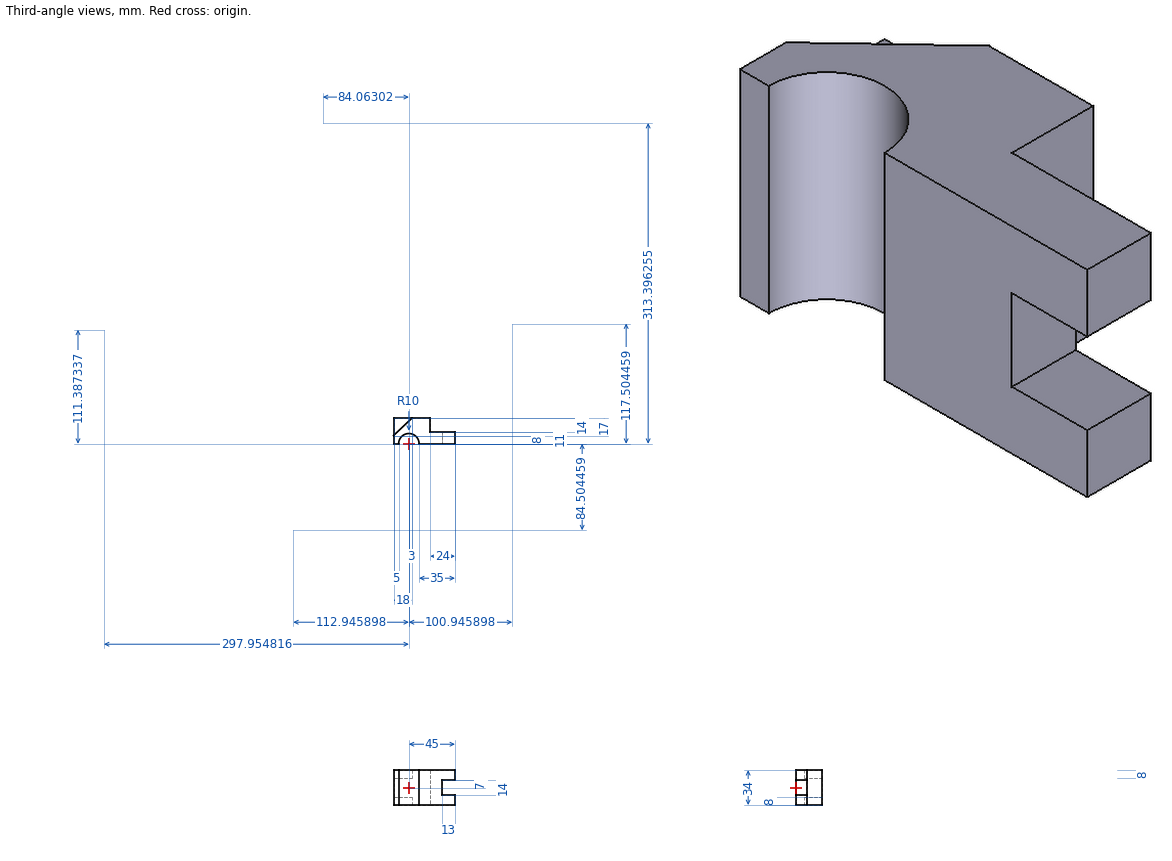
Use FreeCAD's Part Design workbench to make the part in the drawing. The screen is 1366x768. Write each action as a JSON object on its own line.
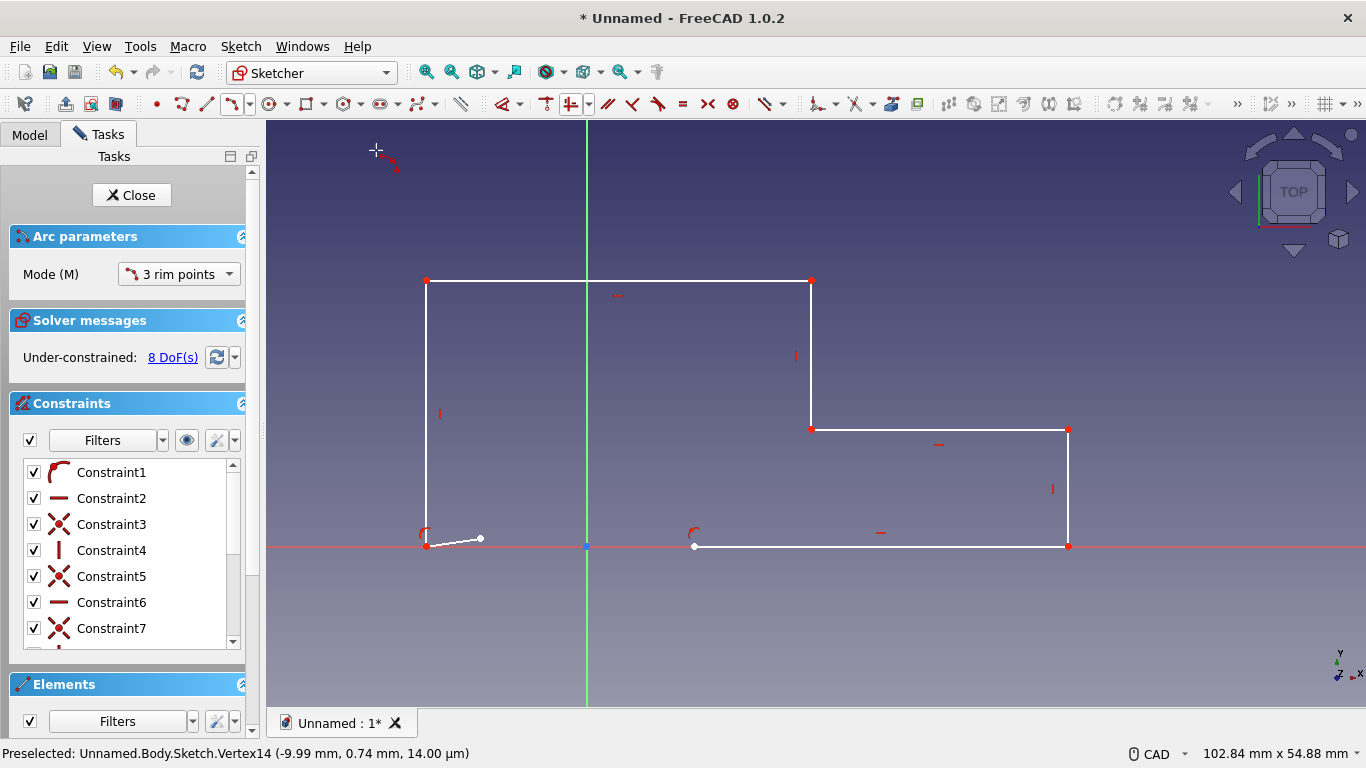
{"action": "left_click", "coordinate": [480, 539]}
{"action": "left_click", "coordinate": [694, 547]}
{"action": "left_click", "coordinate": [620, 445]}
{"action": "key", "text": "Escape"}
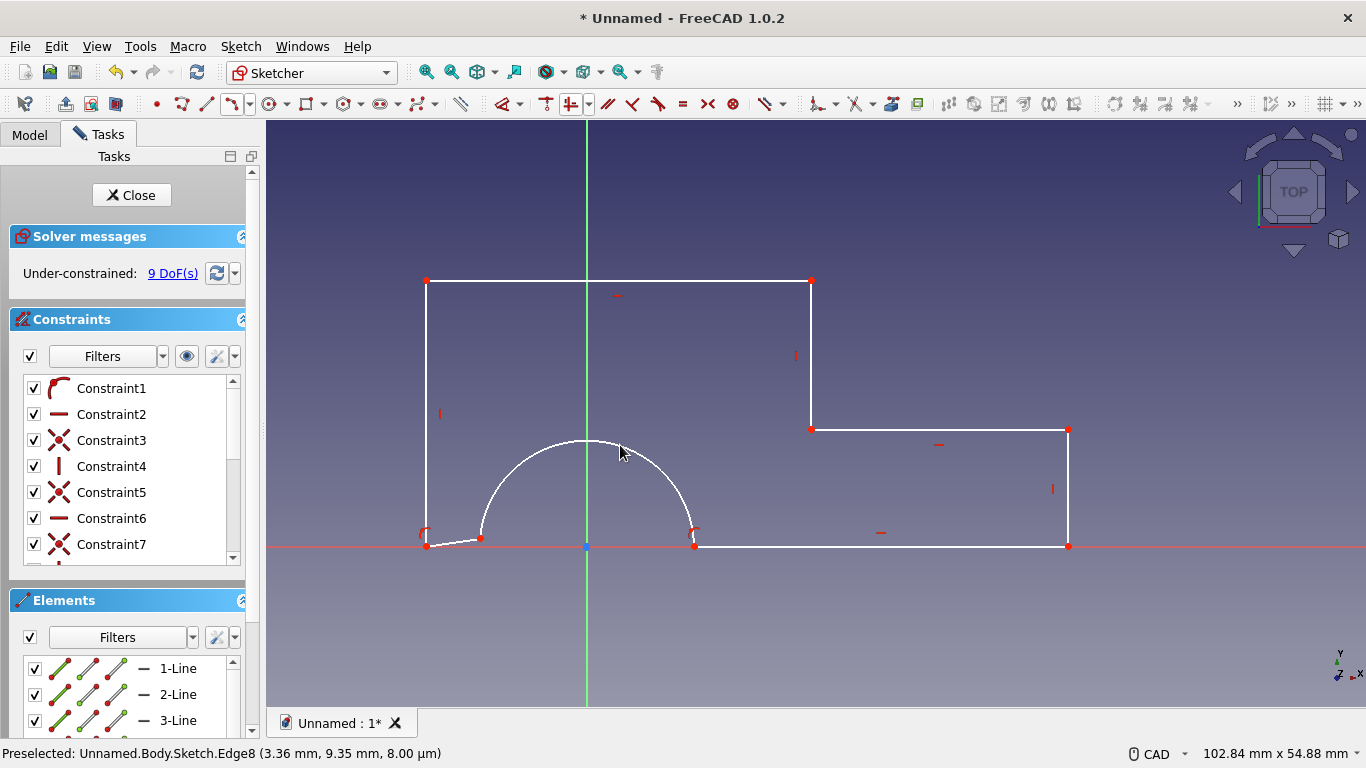
{"action": "left_click", "coordinate": [442, 545]}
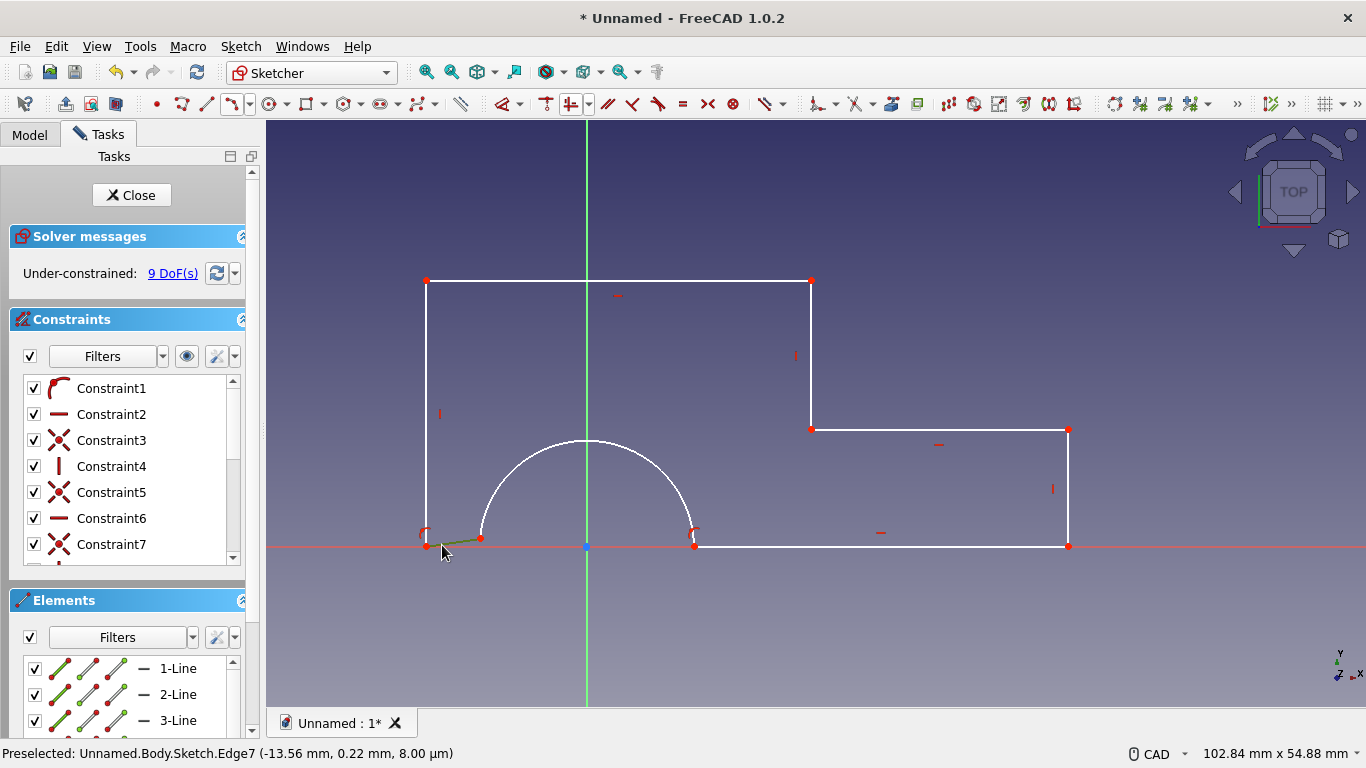
{"action": "key", "text": "h"}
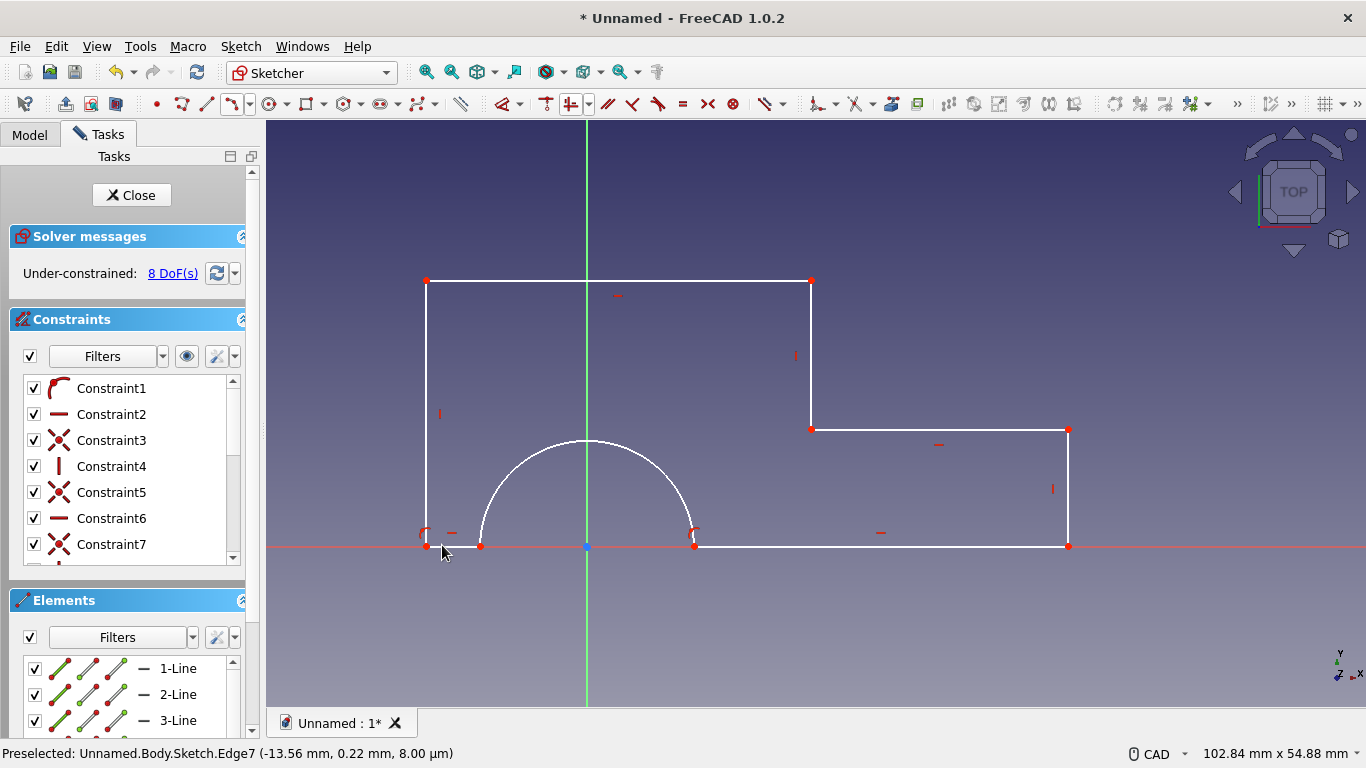
{"action": "left_click_drag", "start_coordinate": [577, 537], "coordinate": [597, 558]}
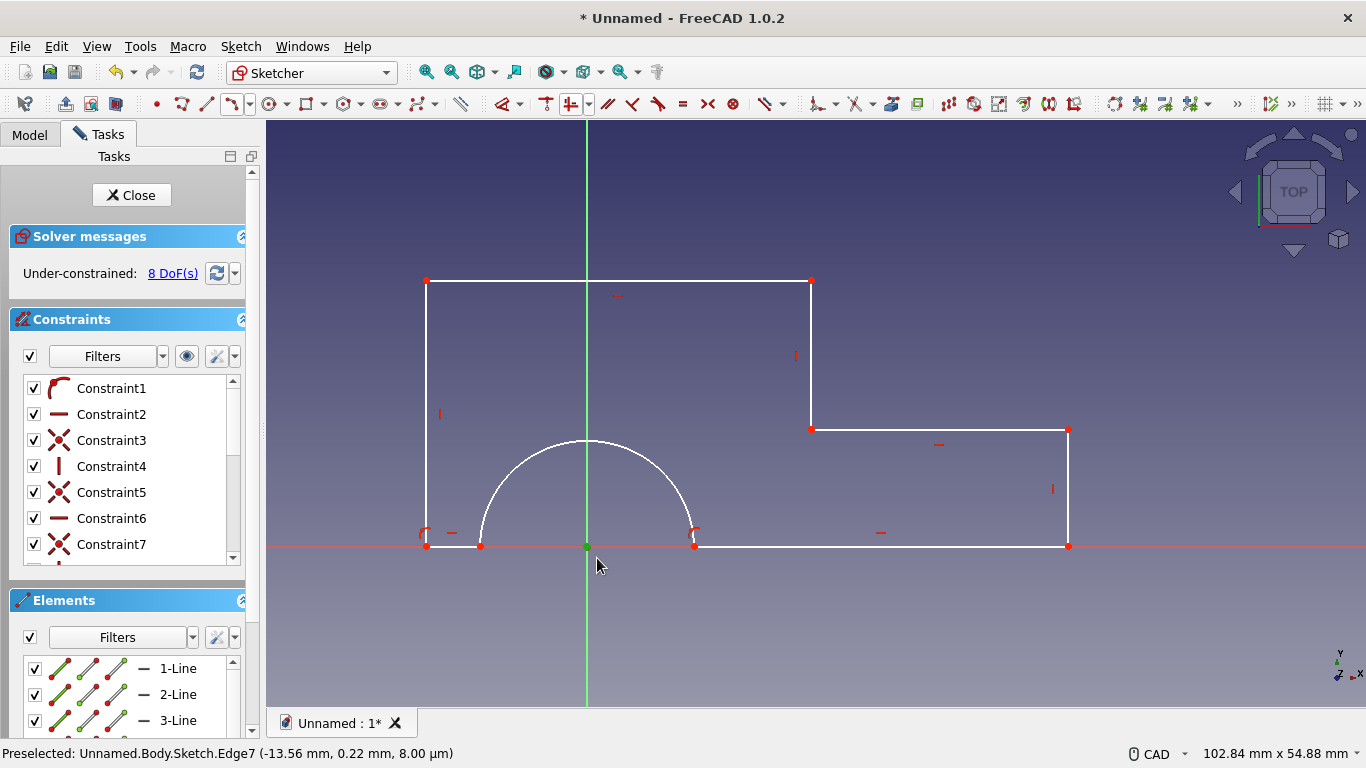
{"action": "left_click", "coordinate": [546, 104]}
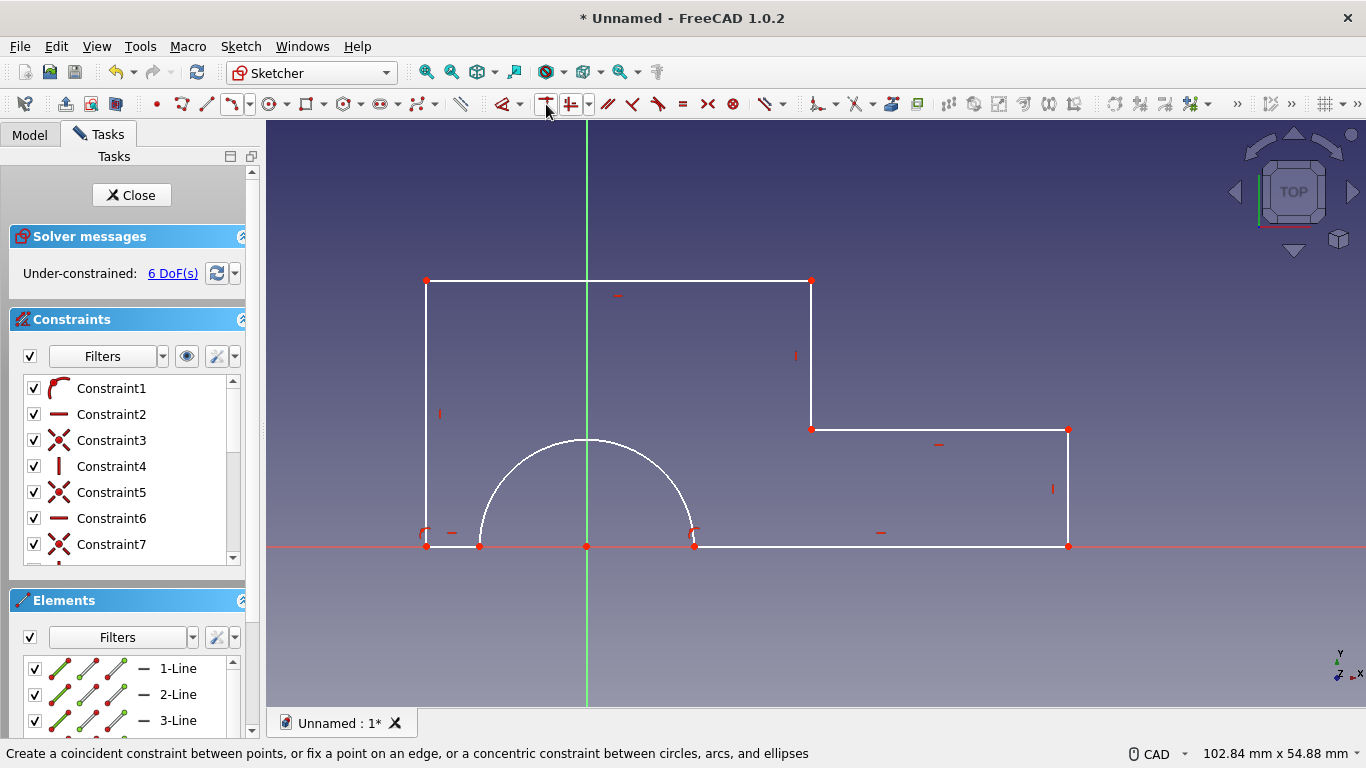
{"action": "left_click", "coordinate": [502, 104]}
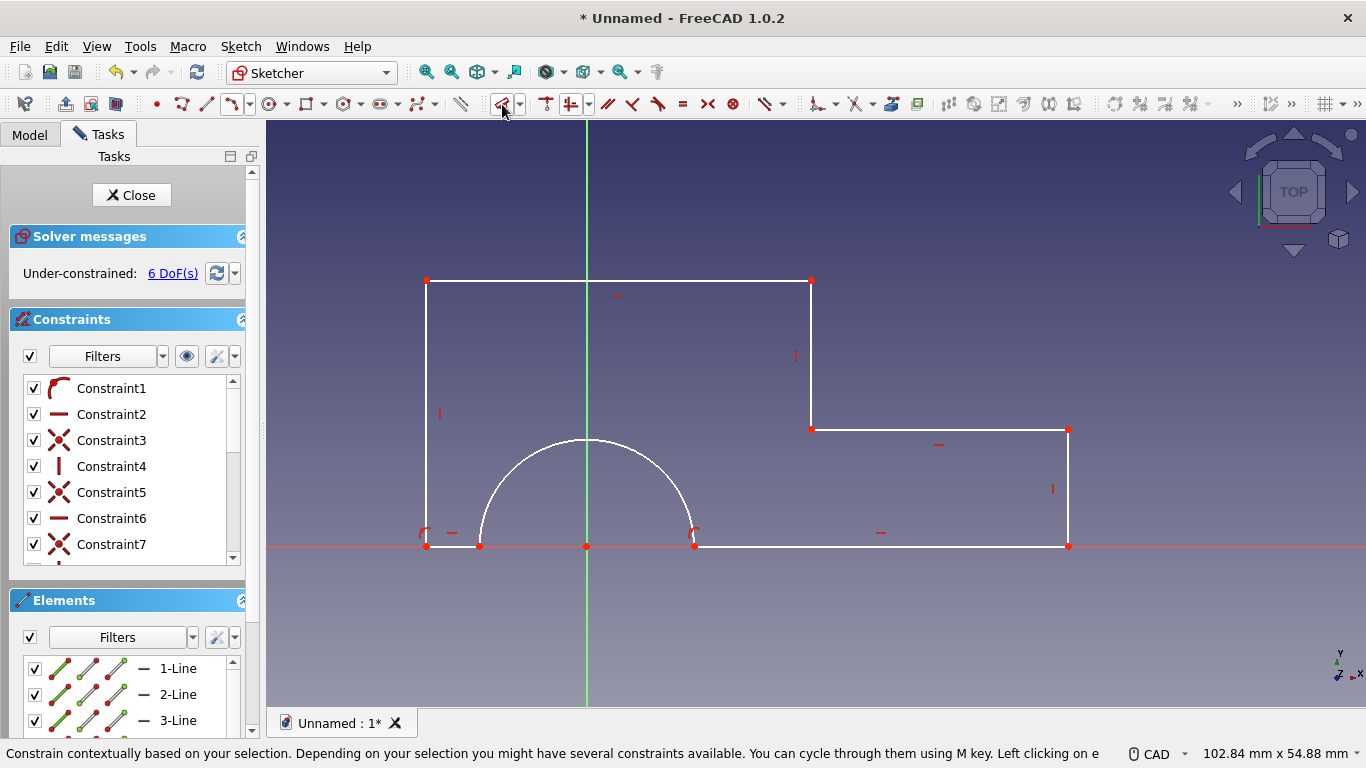
{"action": "left_click", "coordinate": [650, 460]}
{"action": "left_click", "coordinate": [669, 434]}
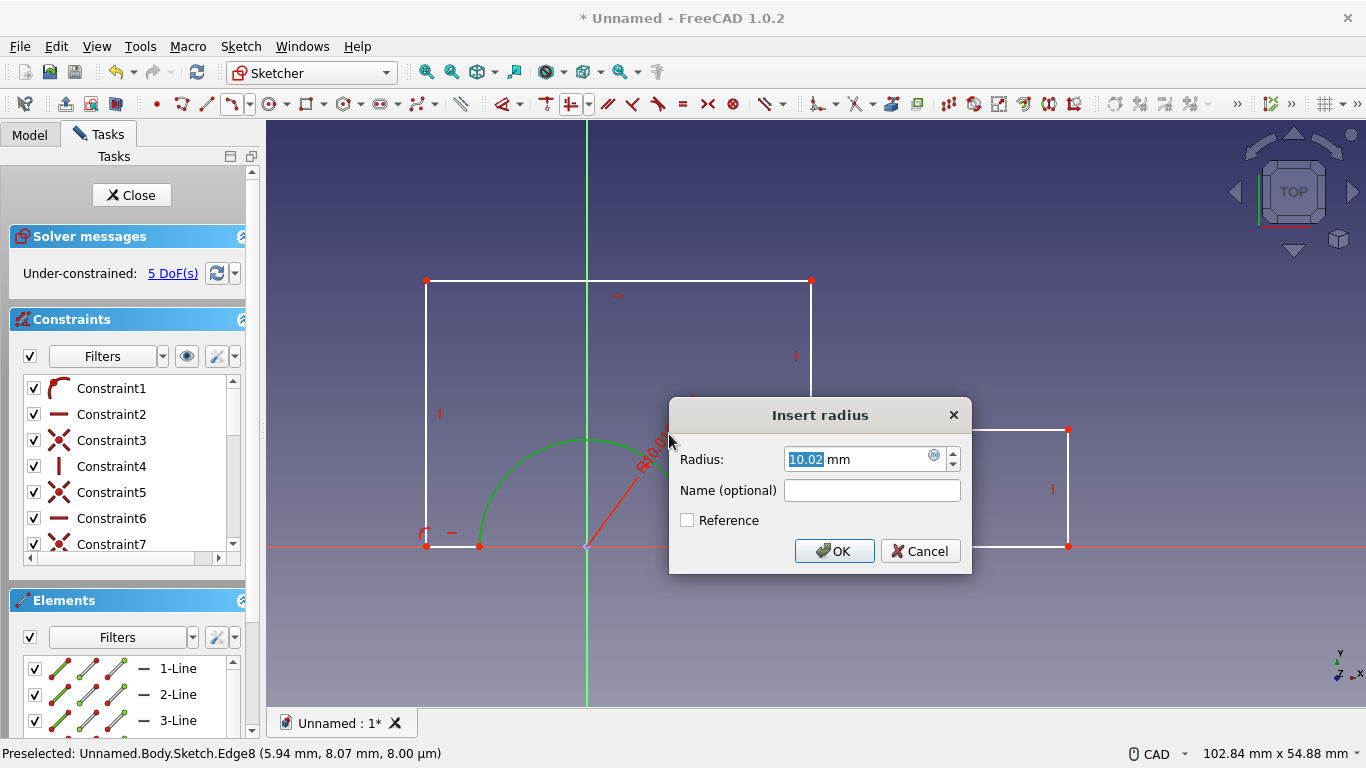
{"action": "type", "text": "10"}
{"action": "key", "text": "Return"}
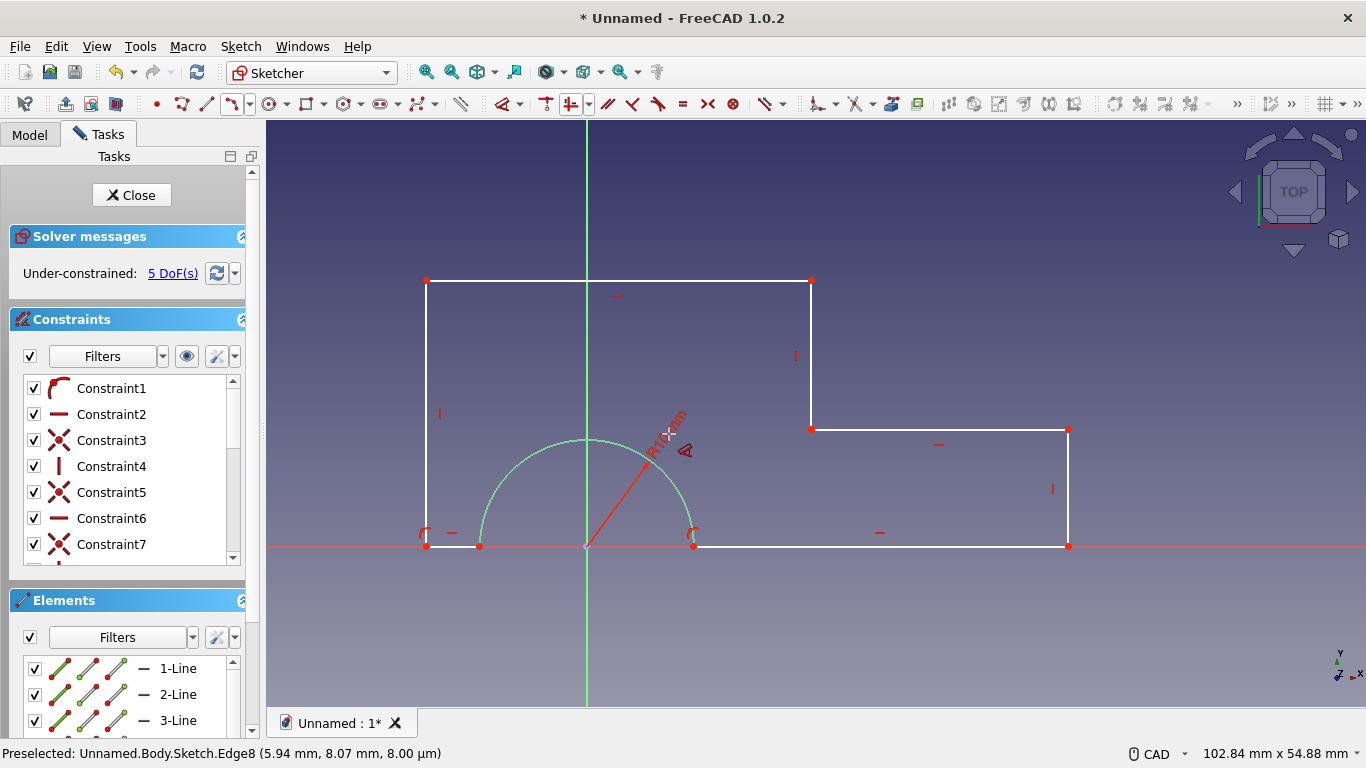
{"action": "left_click", "coordinate": [442, 547]}
{"action": "left_click", "coordinate": [453, 581]}